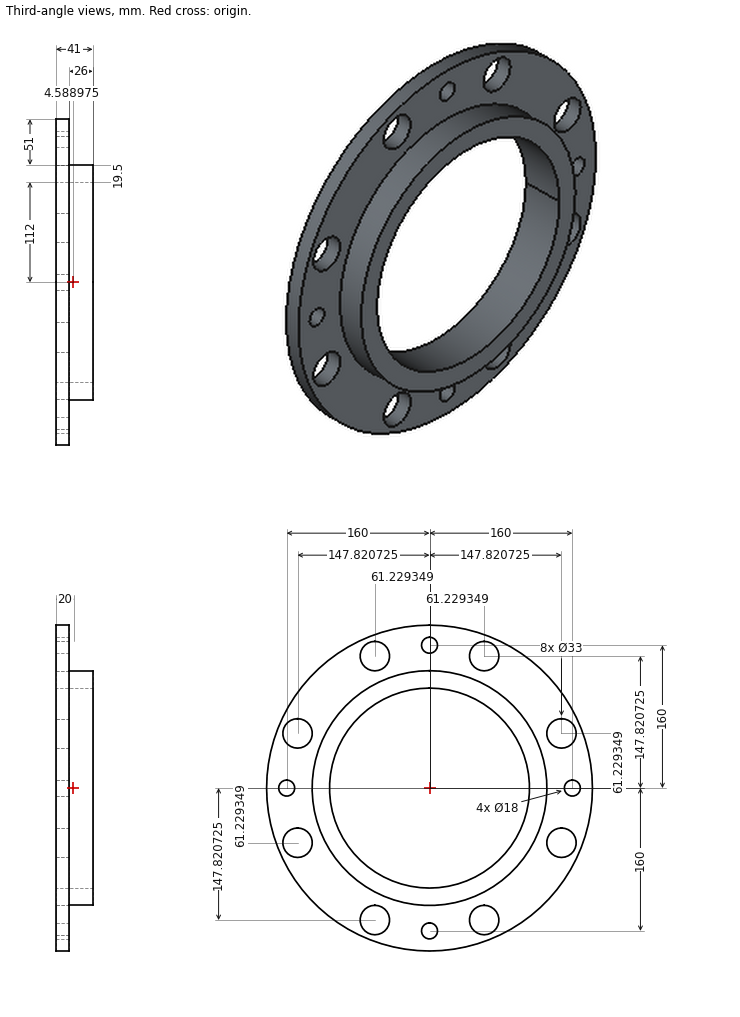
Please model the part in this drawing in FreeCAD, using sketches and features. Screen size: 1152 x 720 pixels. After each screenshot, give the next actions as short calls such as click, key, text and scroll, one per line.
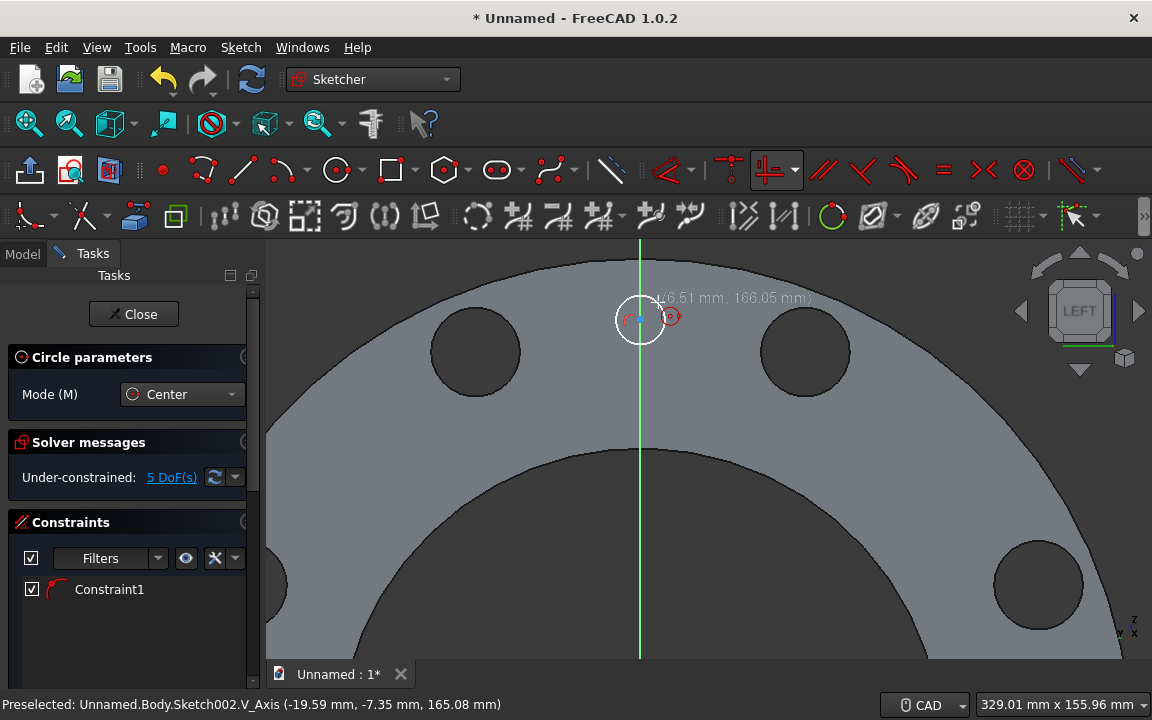
scroll(641, 319, down, 6)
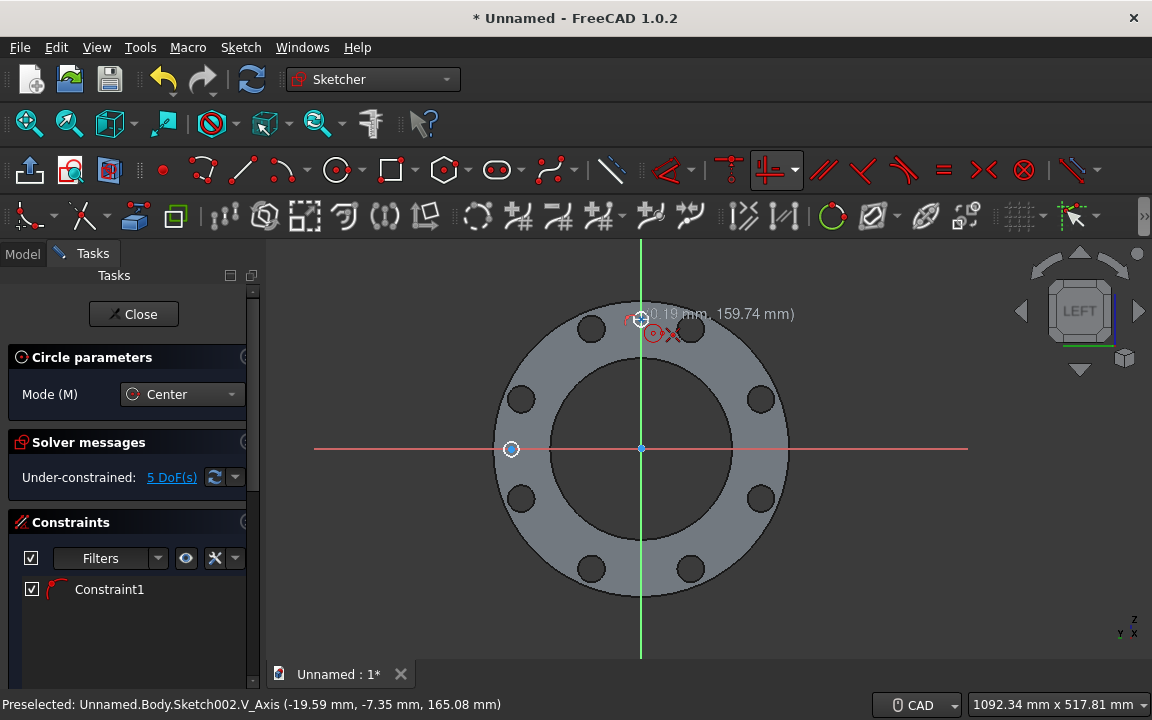
scroll(771, 449, up, 6)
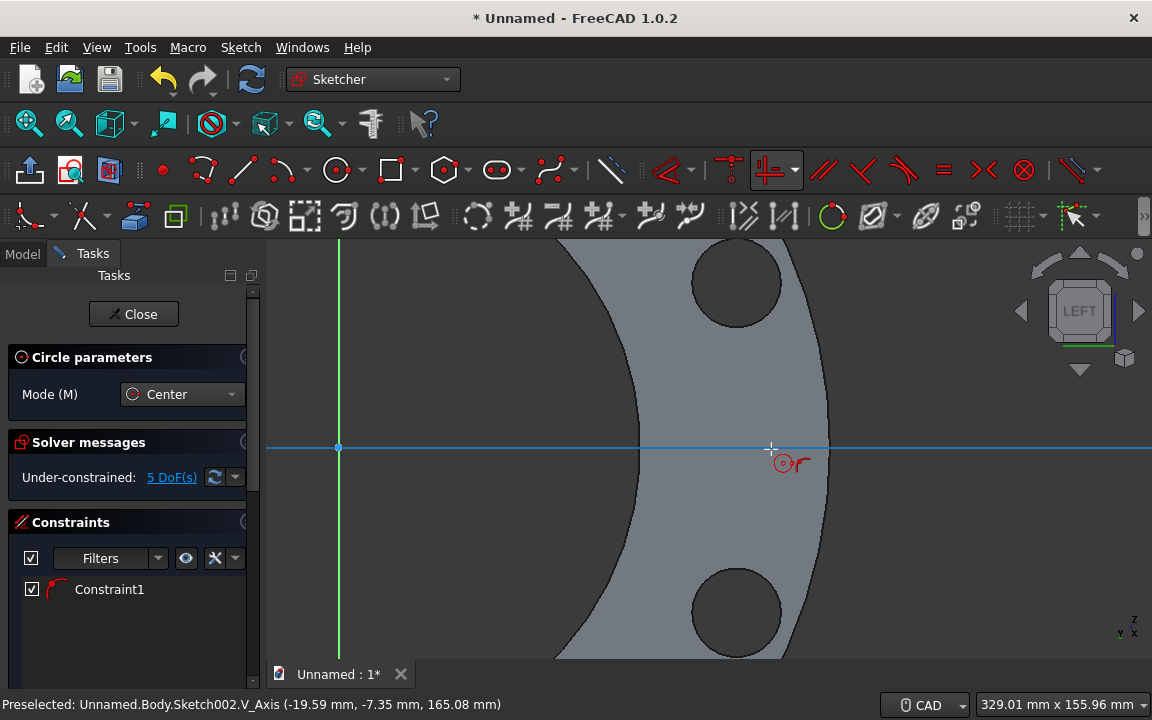
click(769, 448)
click(787, 431)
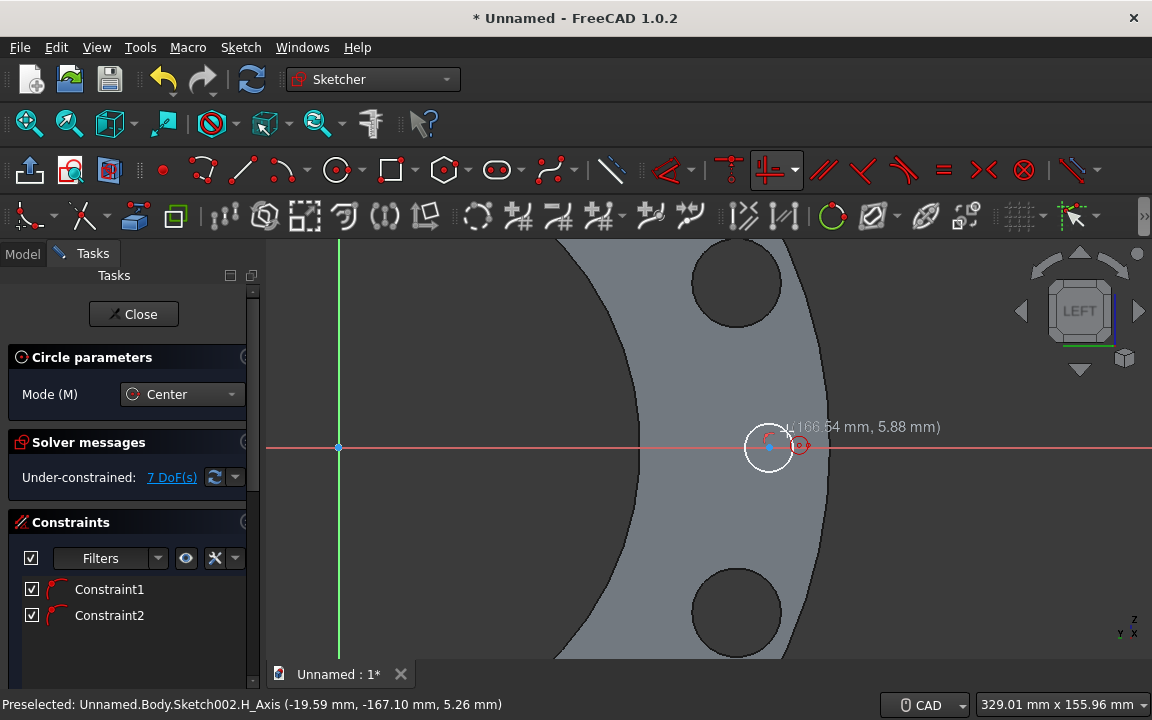
scroll(771, 450, down, 6)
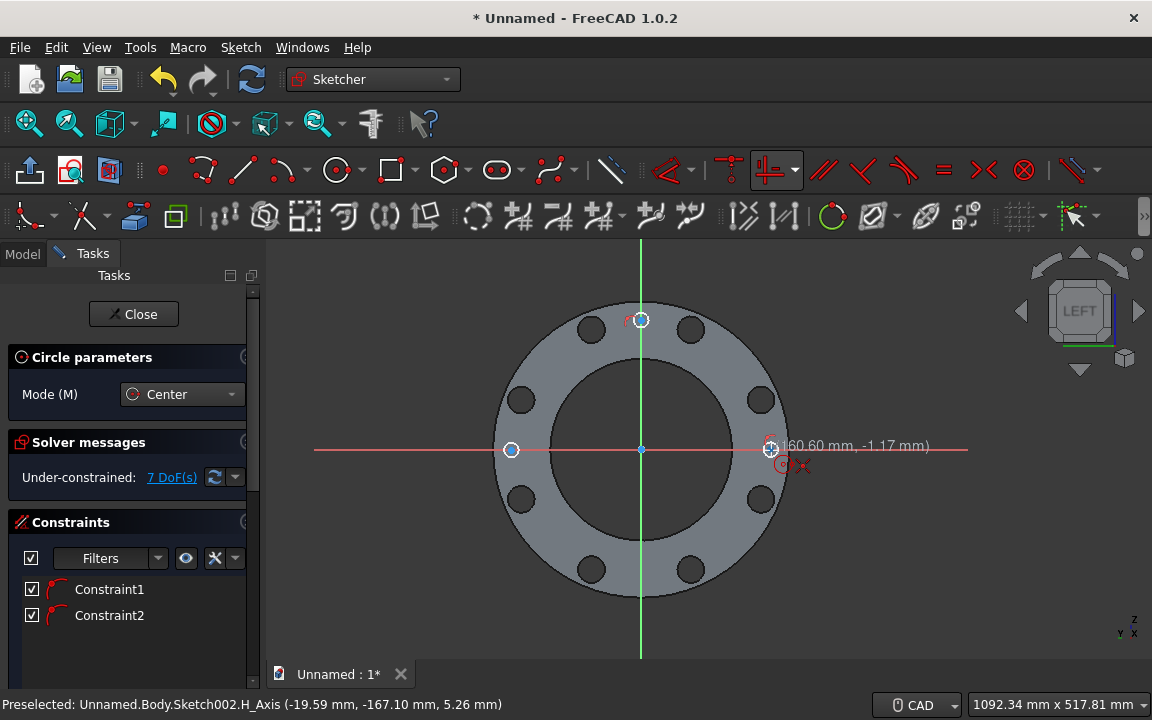
scroll(641, 579, up, 6)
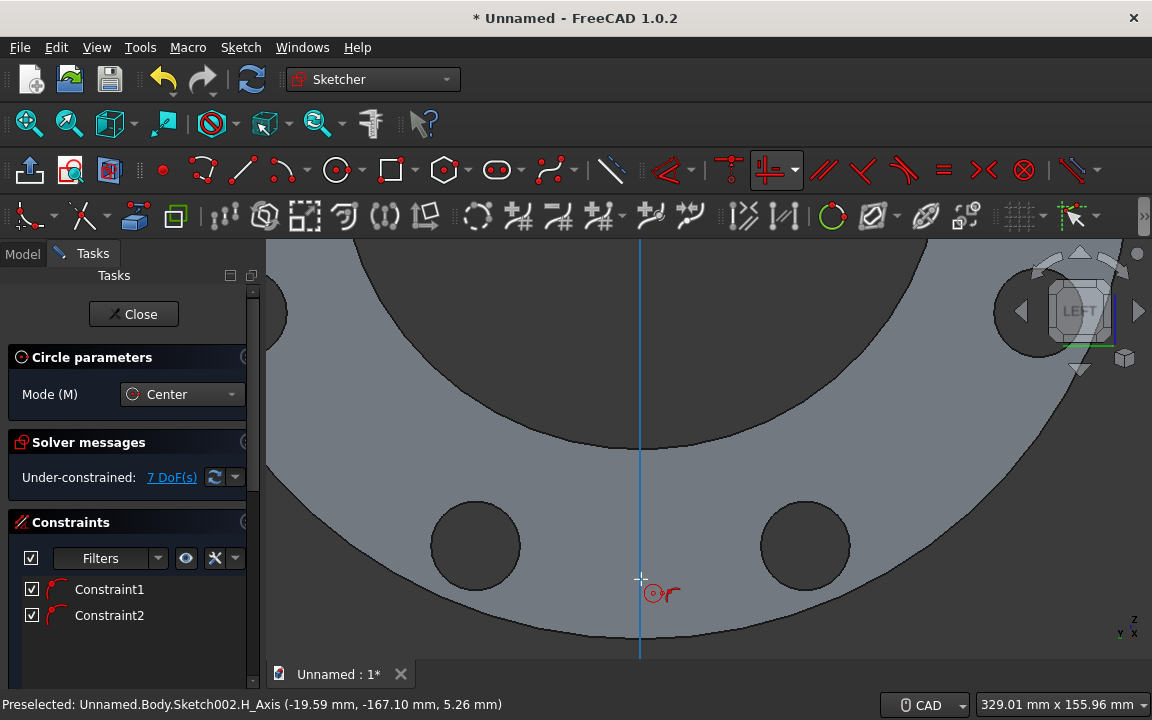
click(640, 579)
click(658, 562)
key(Escape)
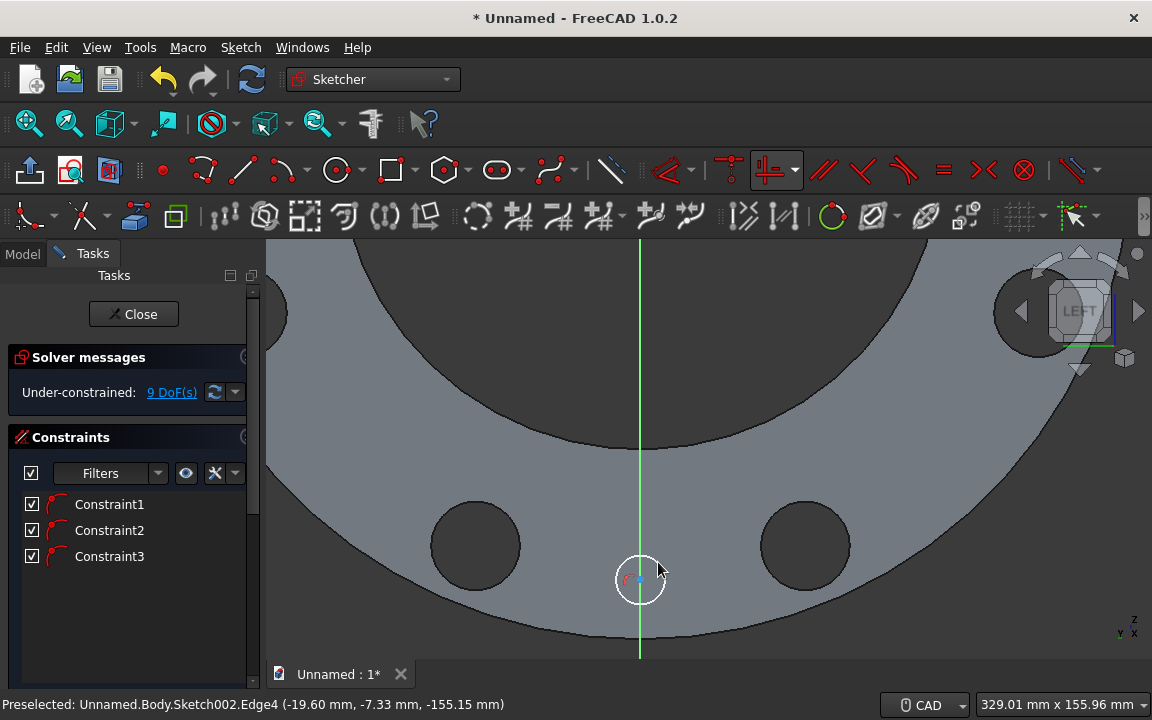
scroll(641, 579, down, 6)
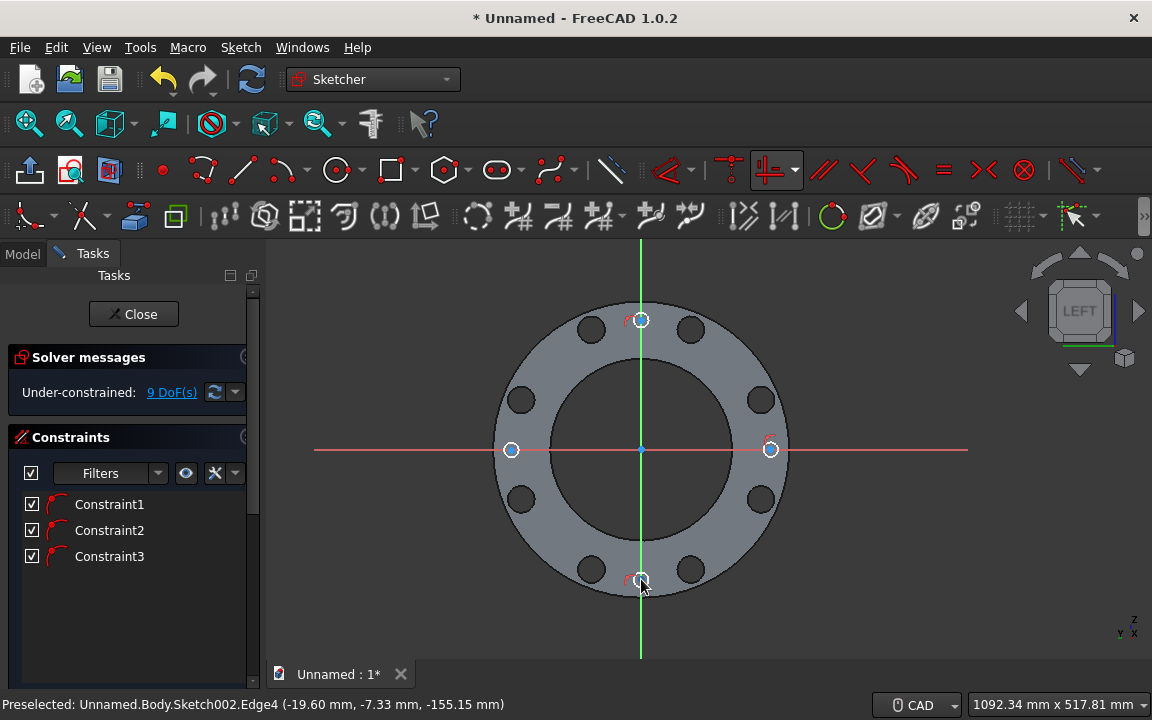
scroll(516, 445, up, 6)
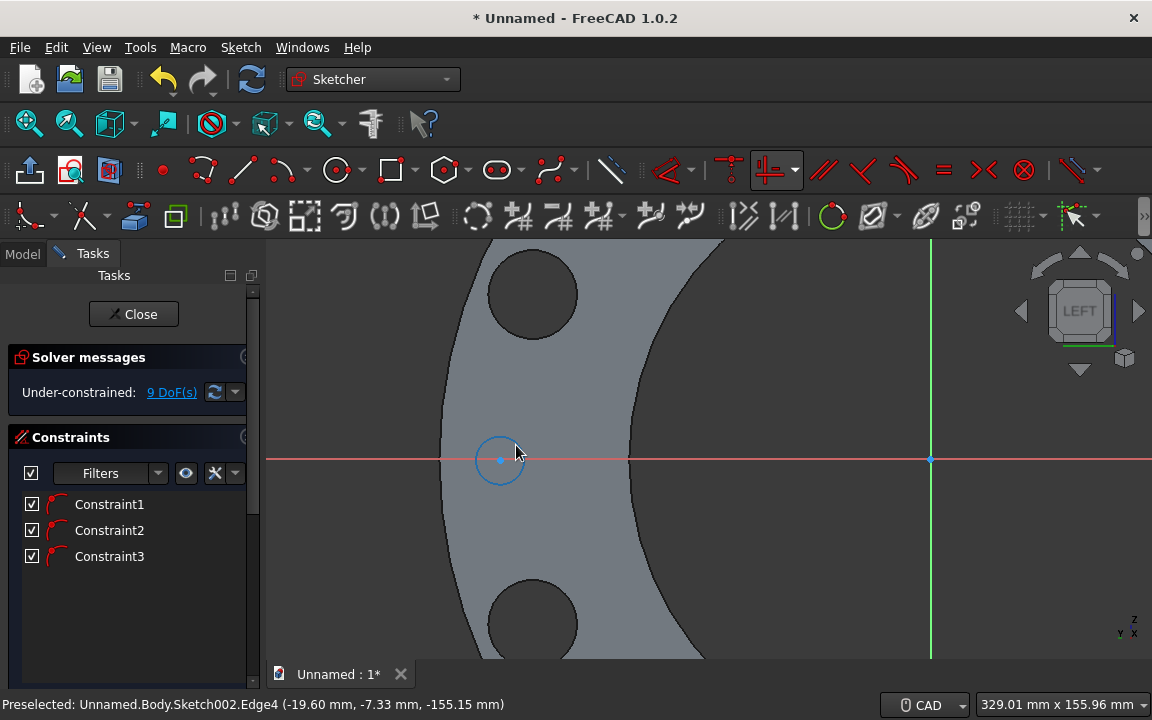
click(517, 444)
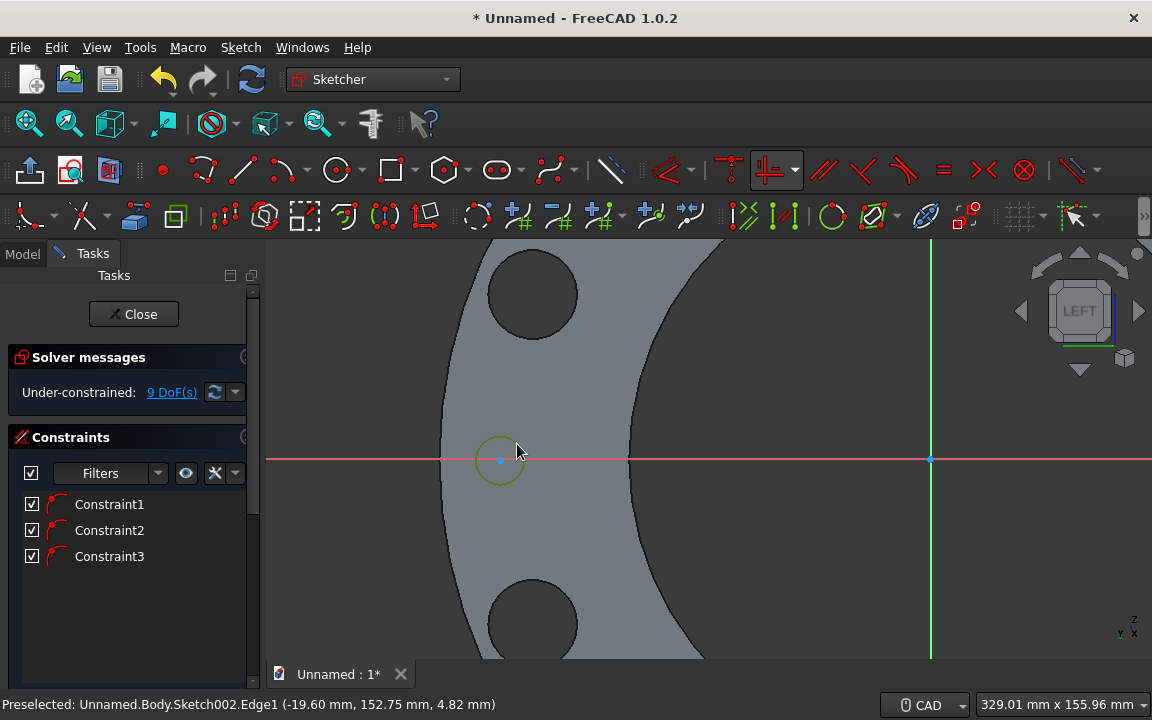
scroll(515, 444, down, 6)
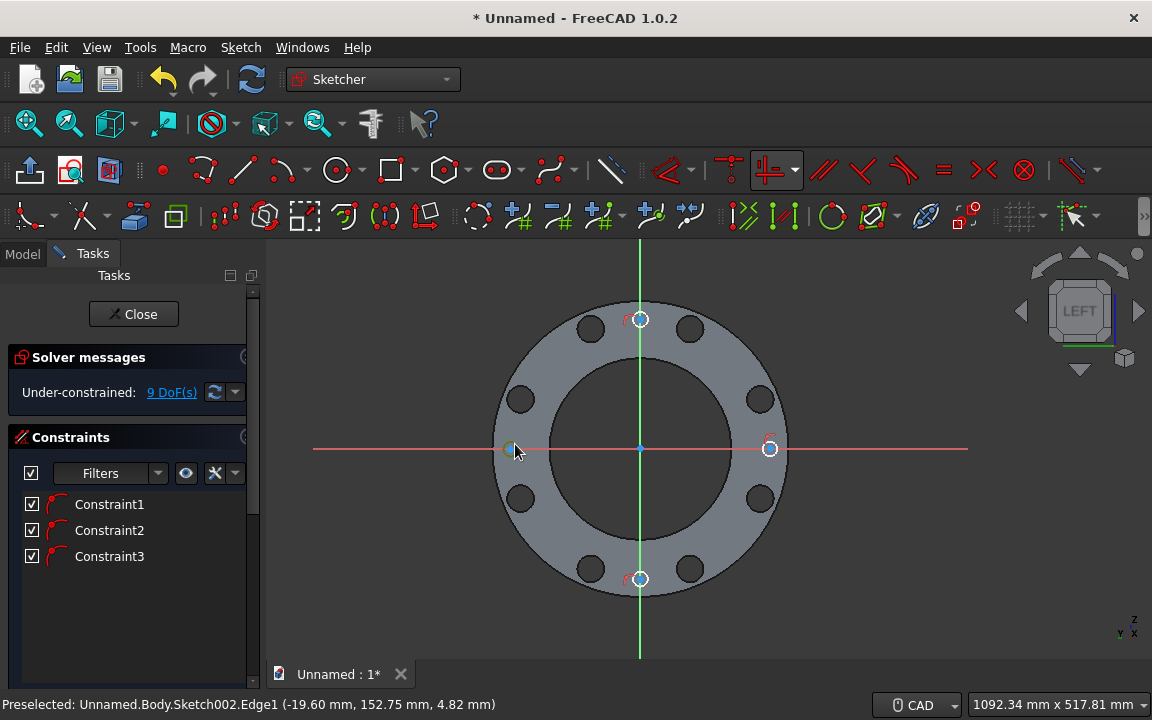
scroll(646, 314, up, 5)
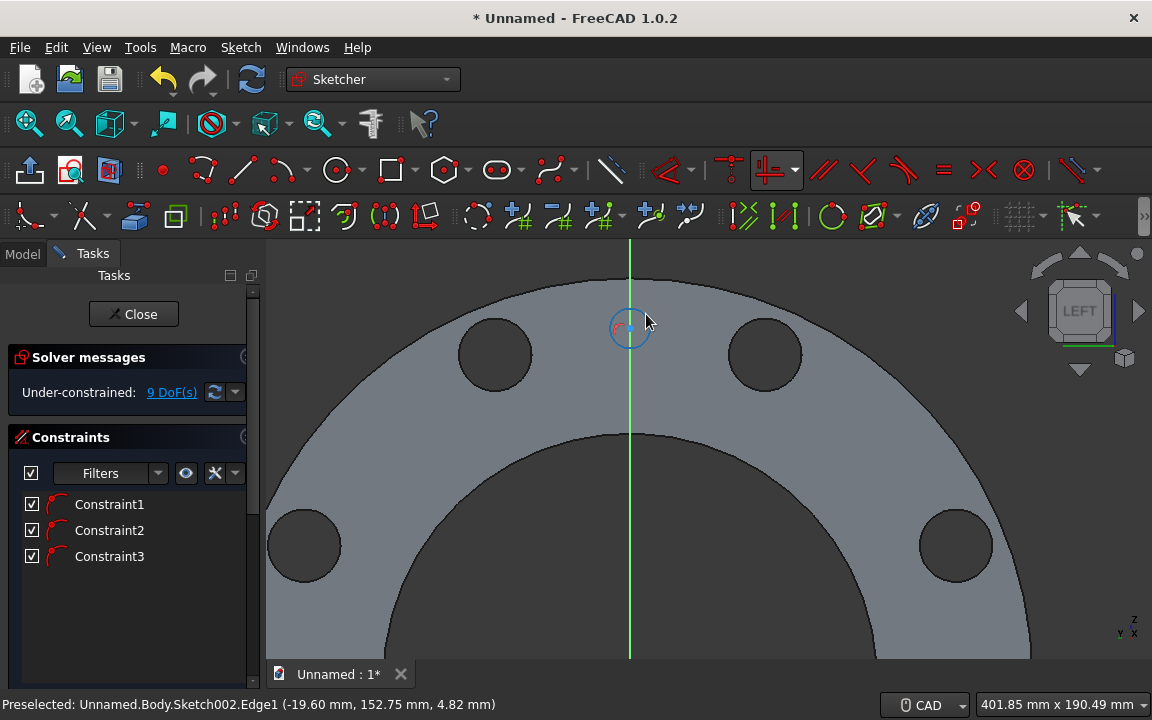
click(644, 314)